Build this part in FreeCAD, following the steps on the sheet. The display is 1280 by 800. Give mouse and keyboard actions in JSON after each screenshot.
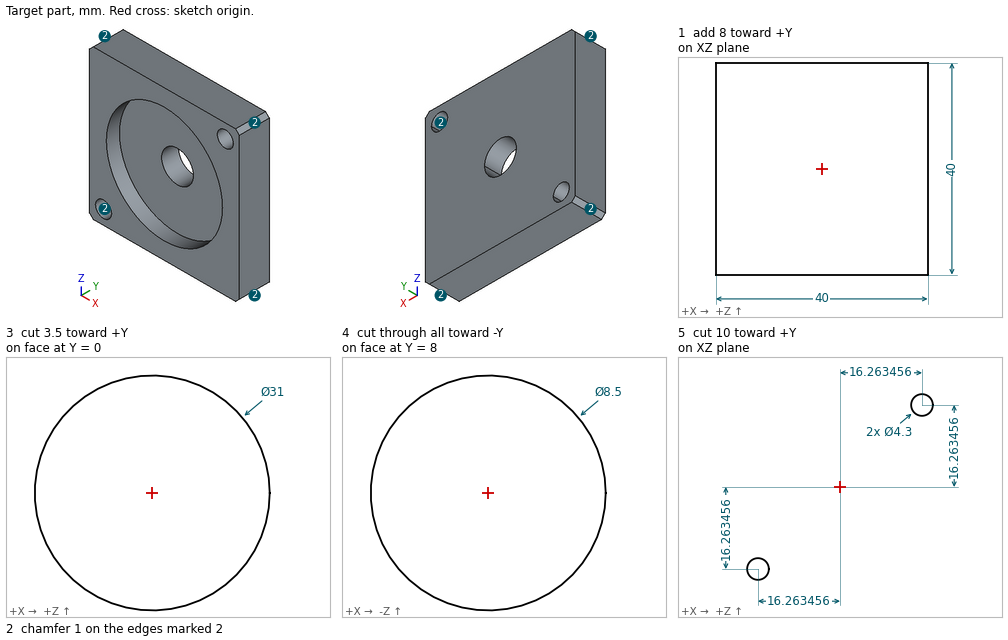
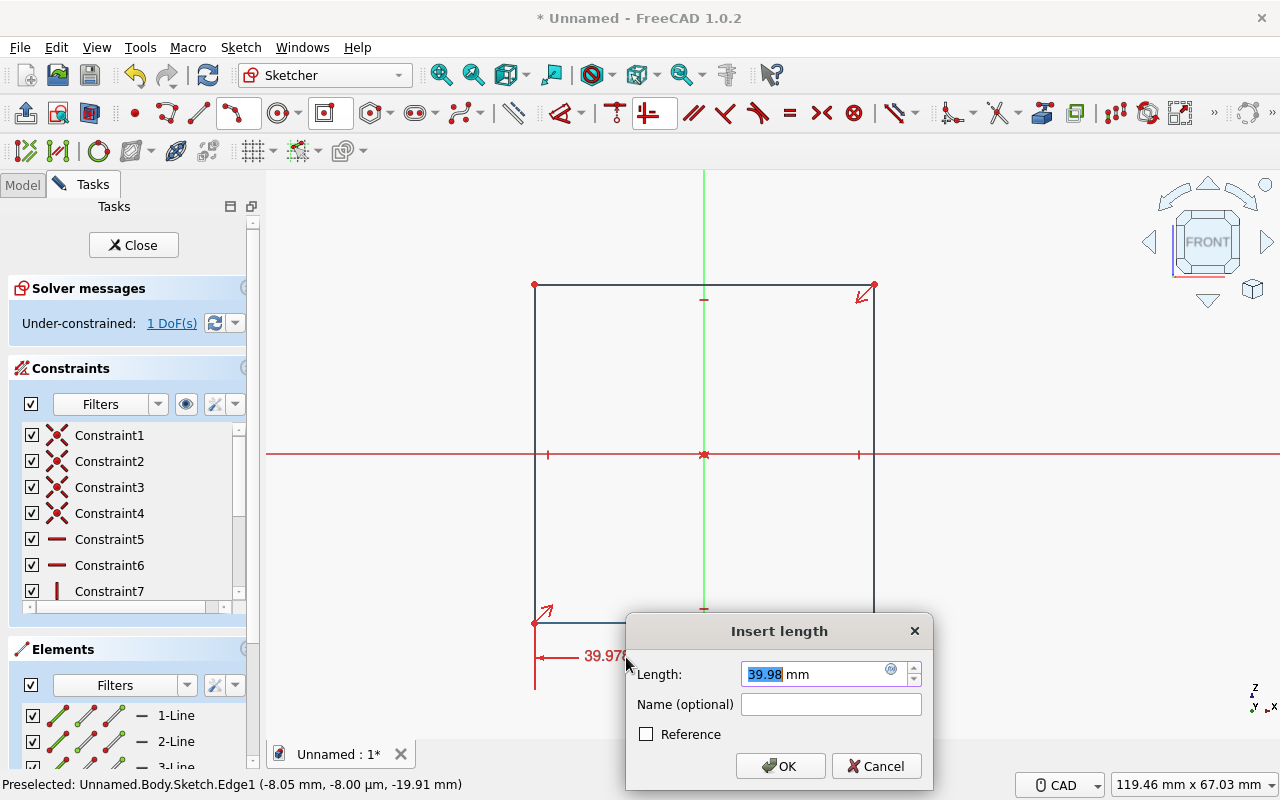
{"action": "type", "text": "40"}
{"action": "key", "text": "Return"}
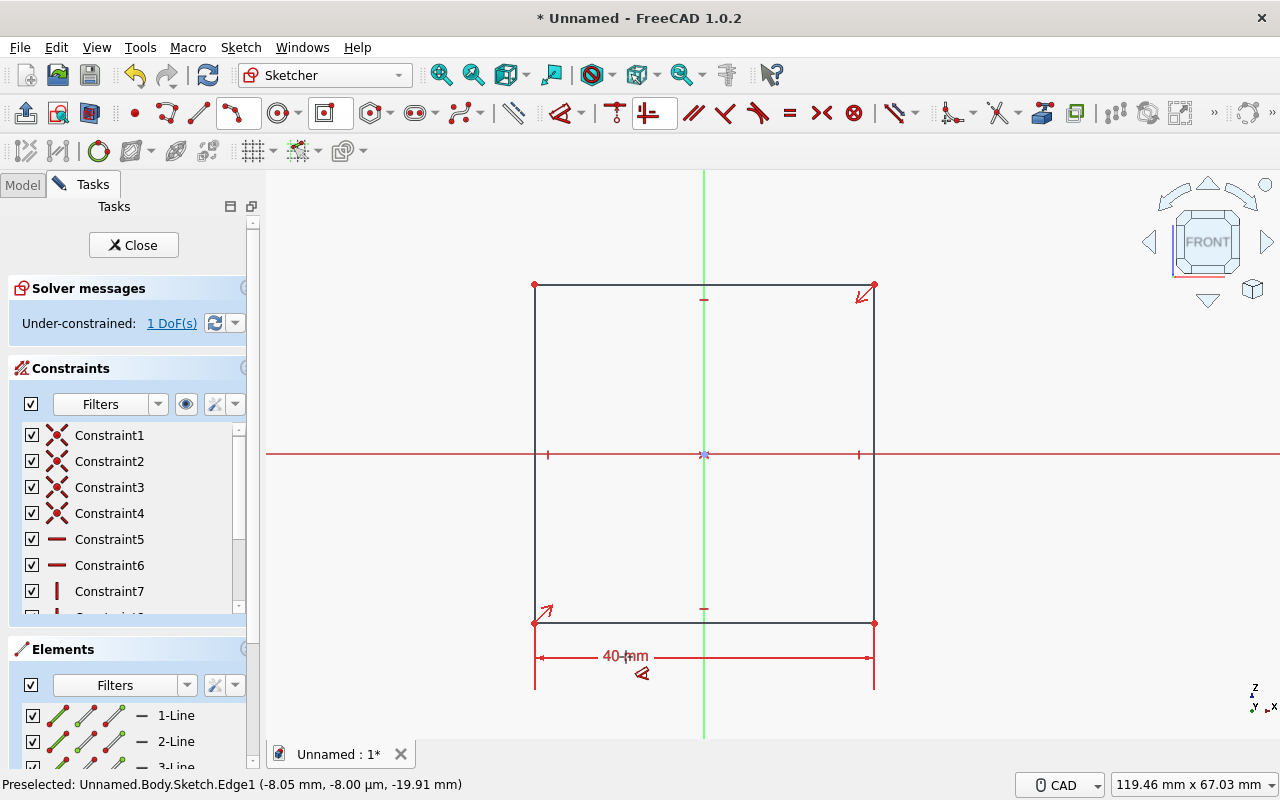
{"action": "left_click", "coordinate": [874, 522]}
{"action": "left_click", "coordinate": [908, 376]}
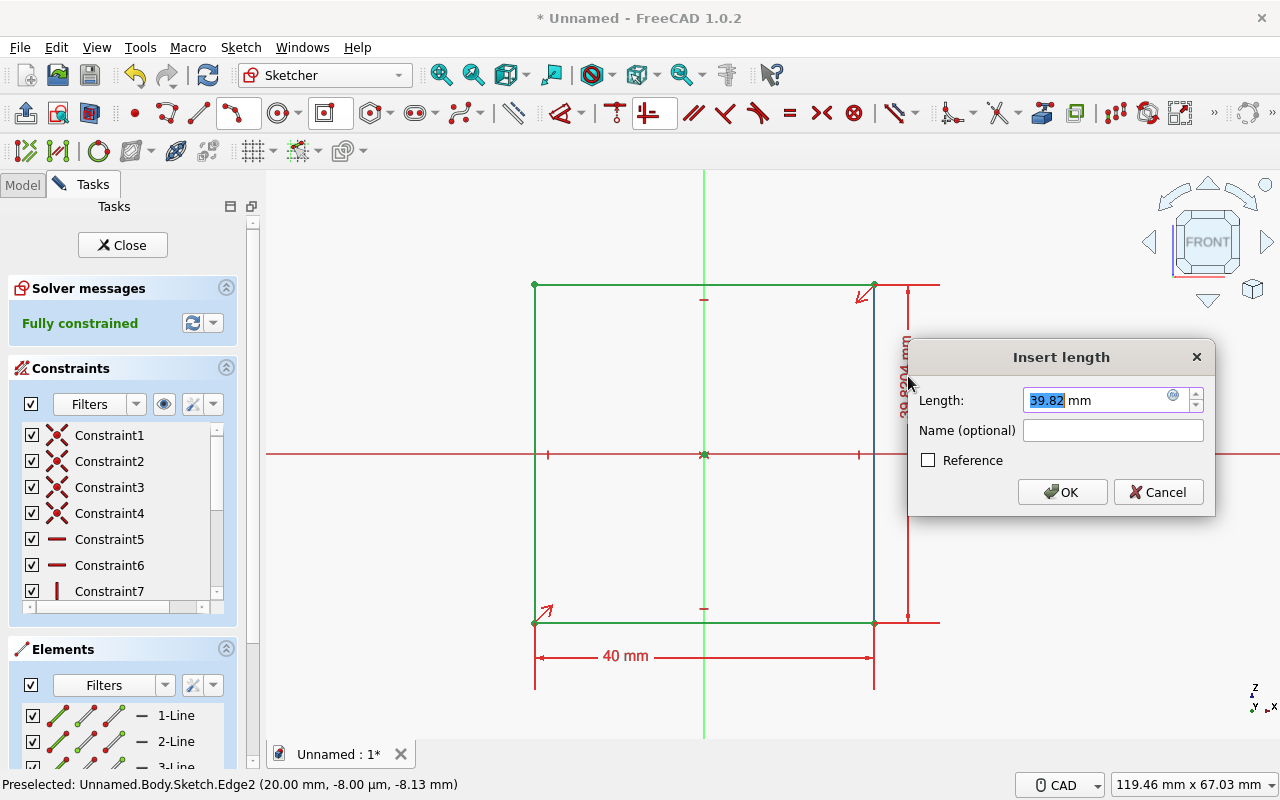
{"action": "type", "text": "40"}
{"action": "key", "text": "Return"}
{"action": "key", "text": "Escape"}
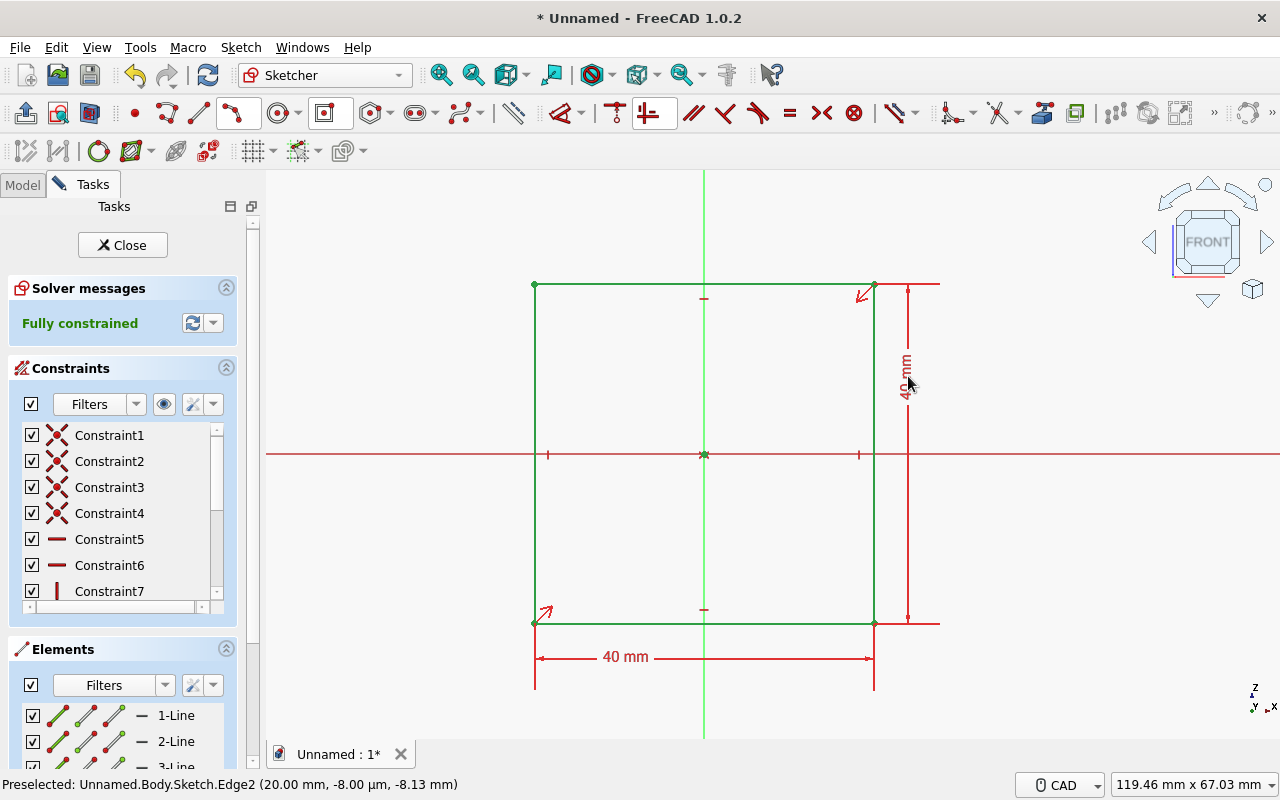
{"action": "left_click", "coordinate": [123, 245]}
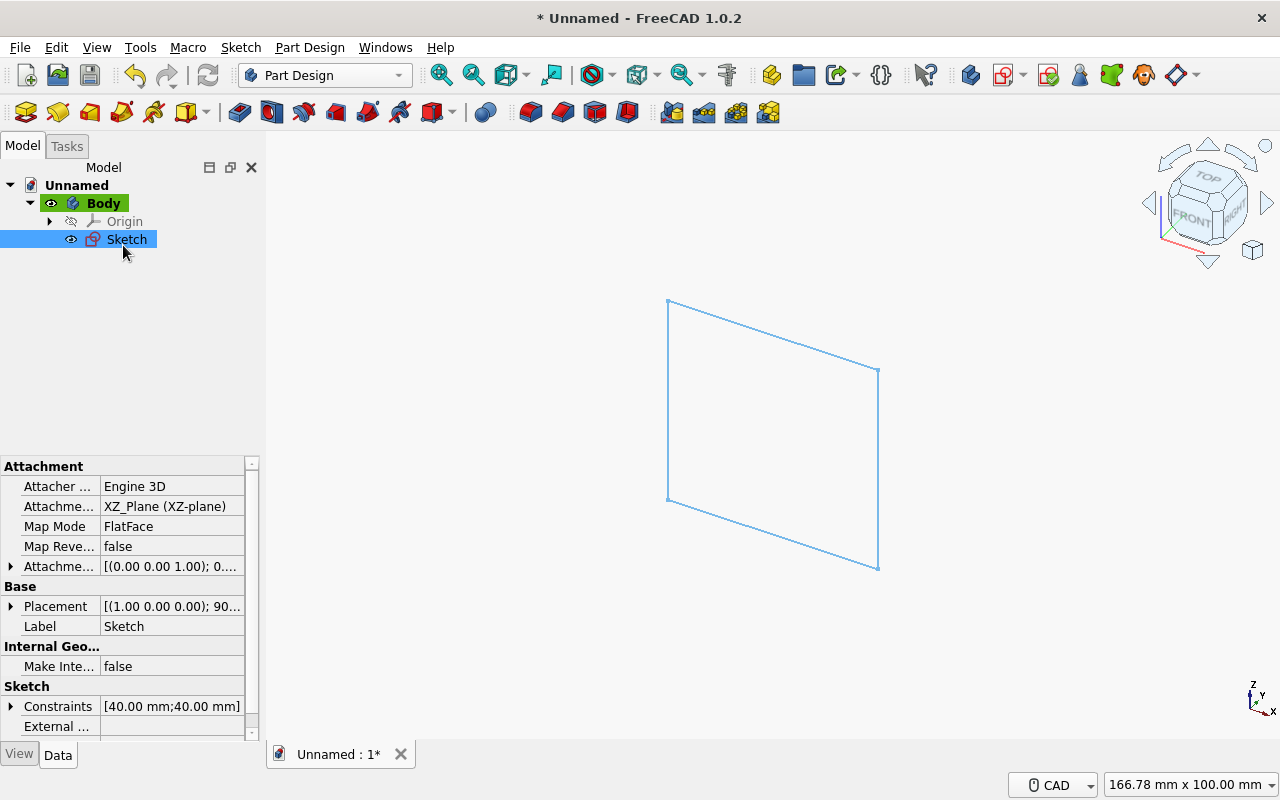
{"action": "left_click", "coordinate": [26, 112]}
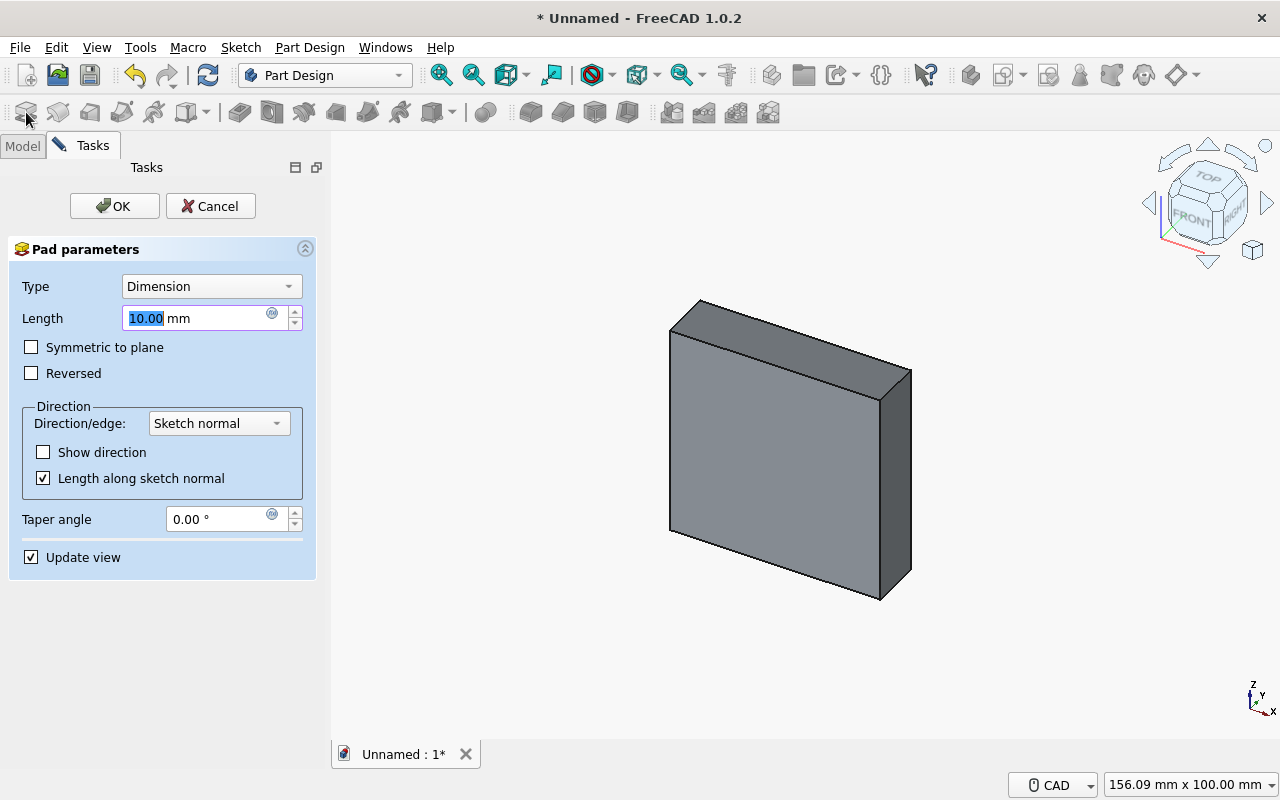
{"action": "type", "text": "8"}
{"action": "key", "text": "Tab"}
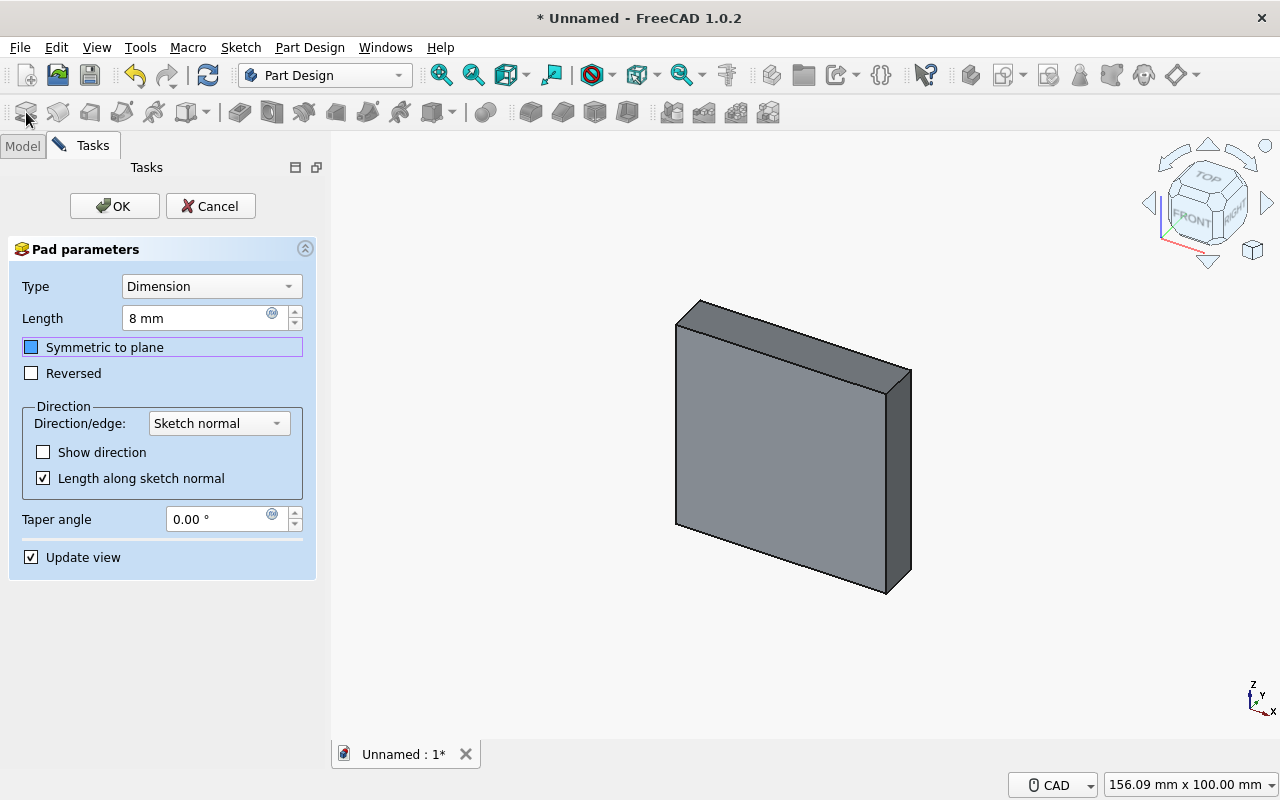
{"action": "left_click", "coordinate": [30, 373]}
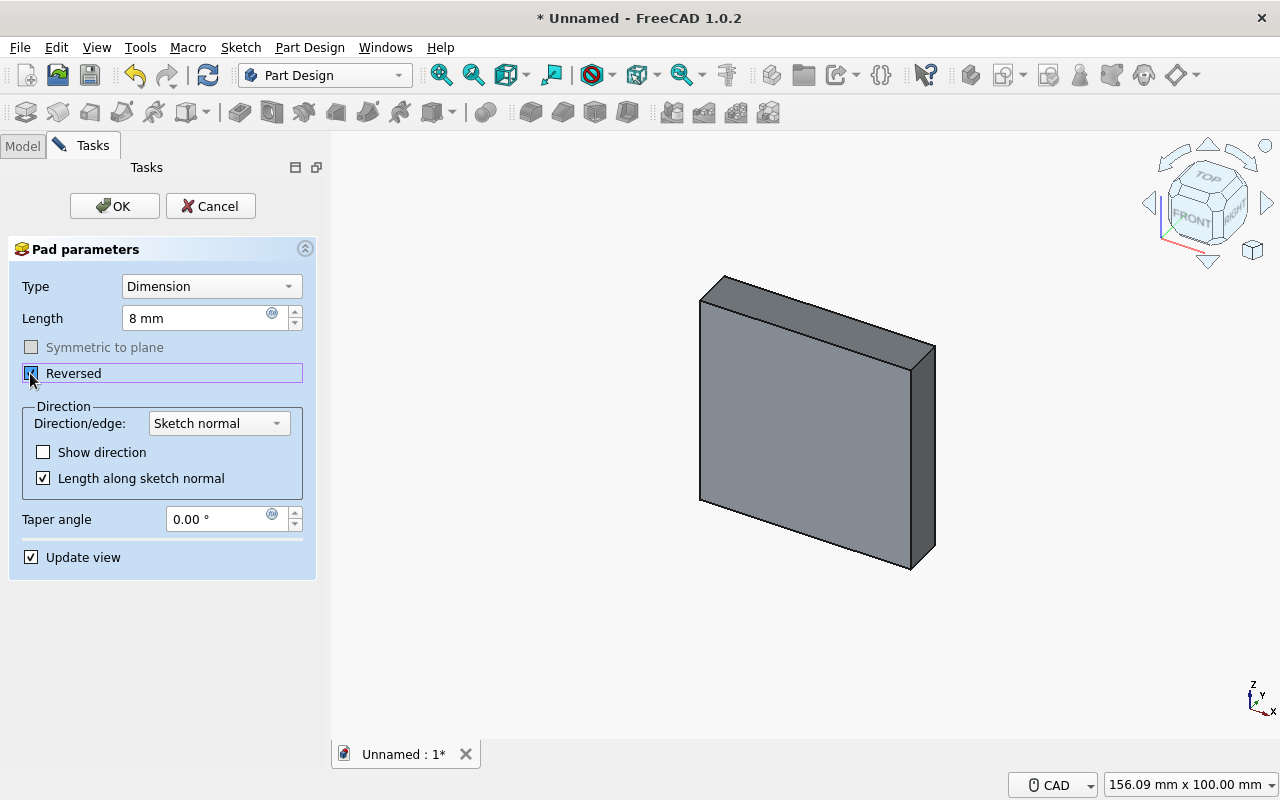
{"action": "left_click", "coordinate": [115, 206]}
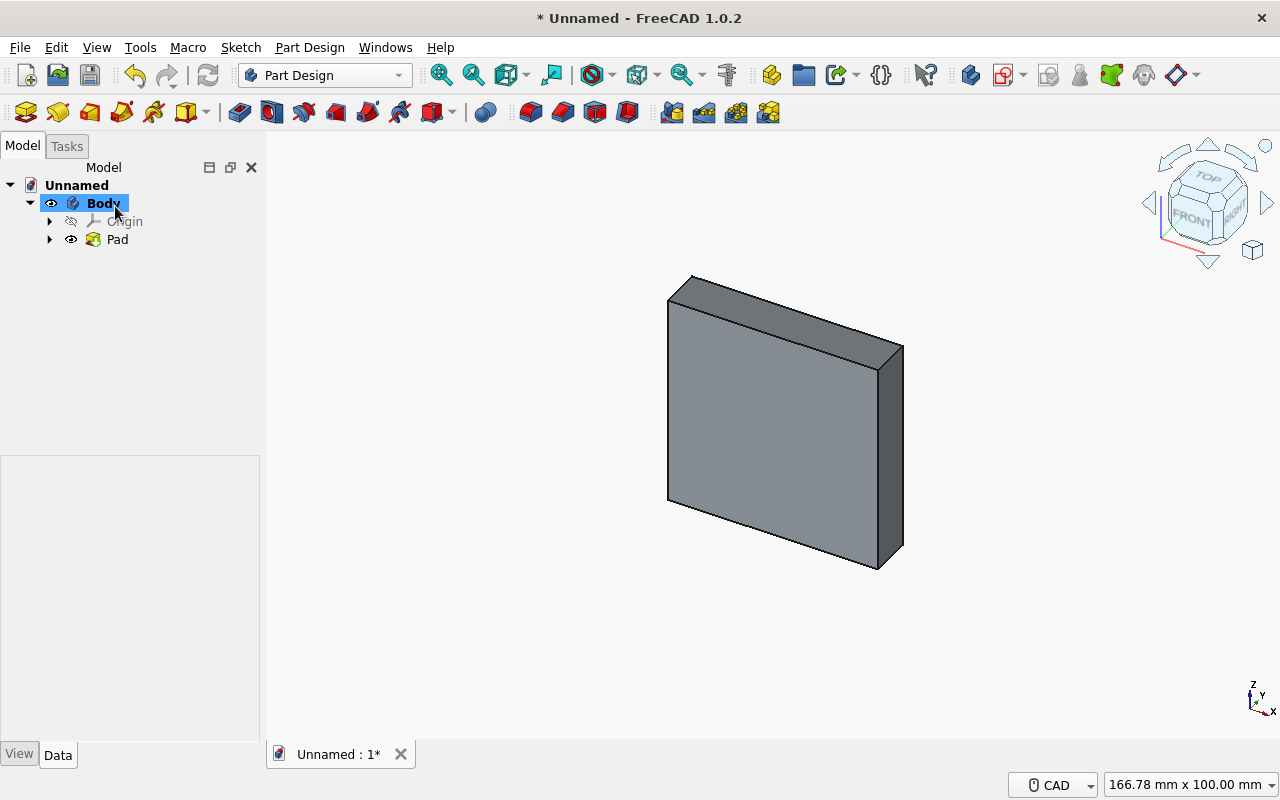
{"action": "left_click", "coordinate": [890, 357]}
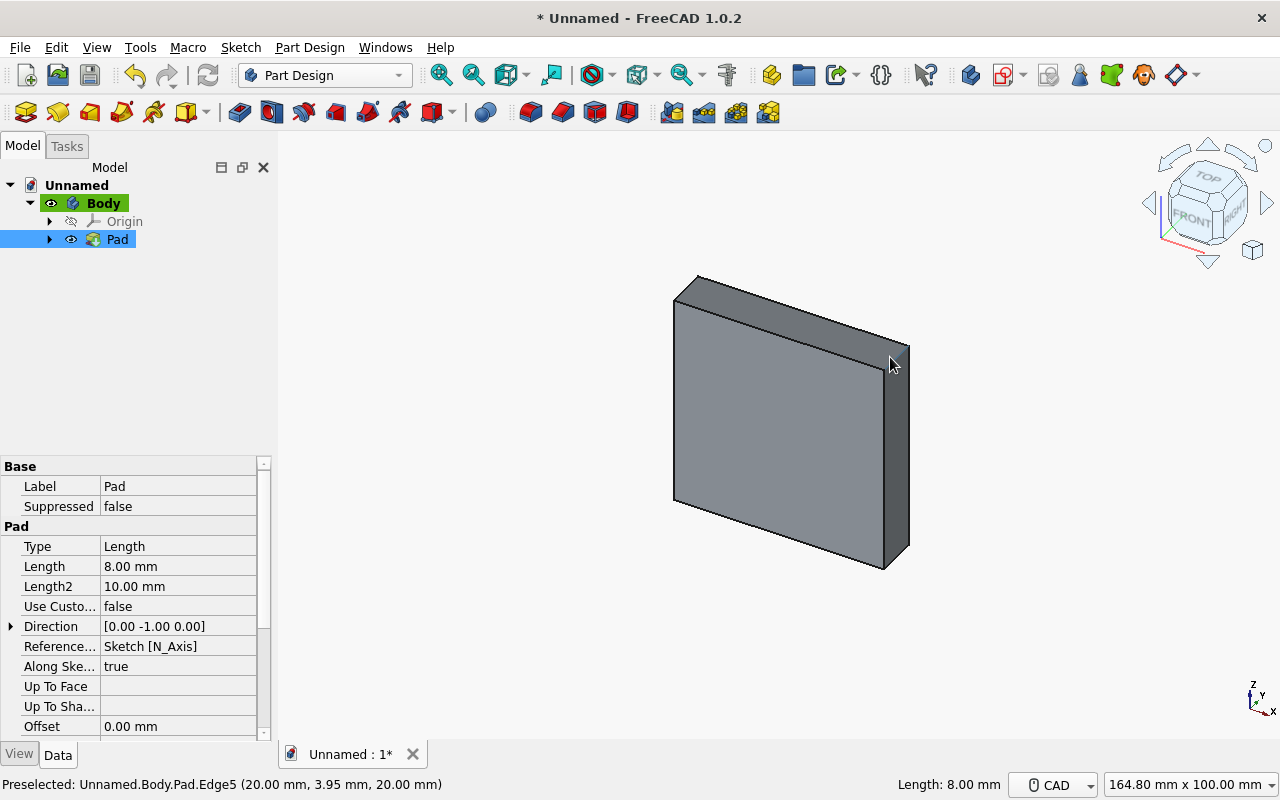
{"action": "key", "text": "0"}